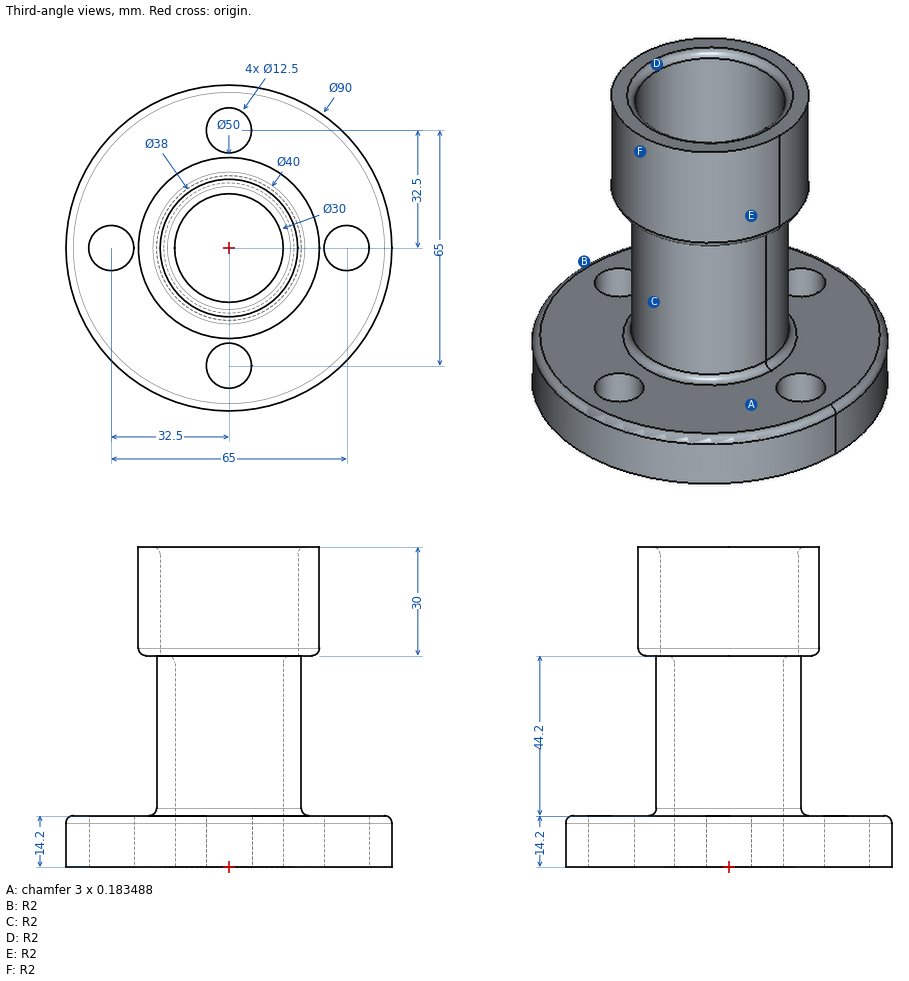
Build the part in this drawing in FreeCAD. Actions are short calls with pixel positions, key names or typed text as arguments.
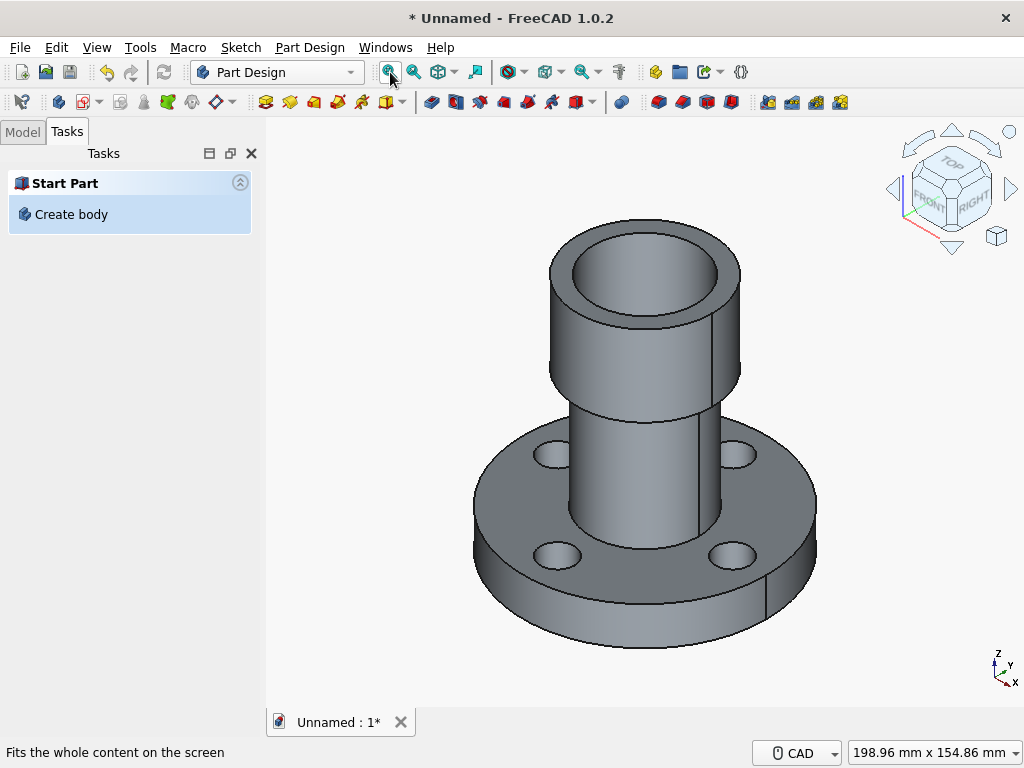
click(492, 549)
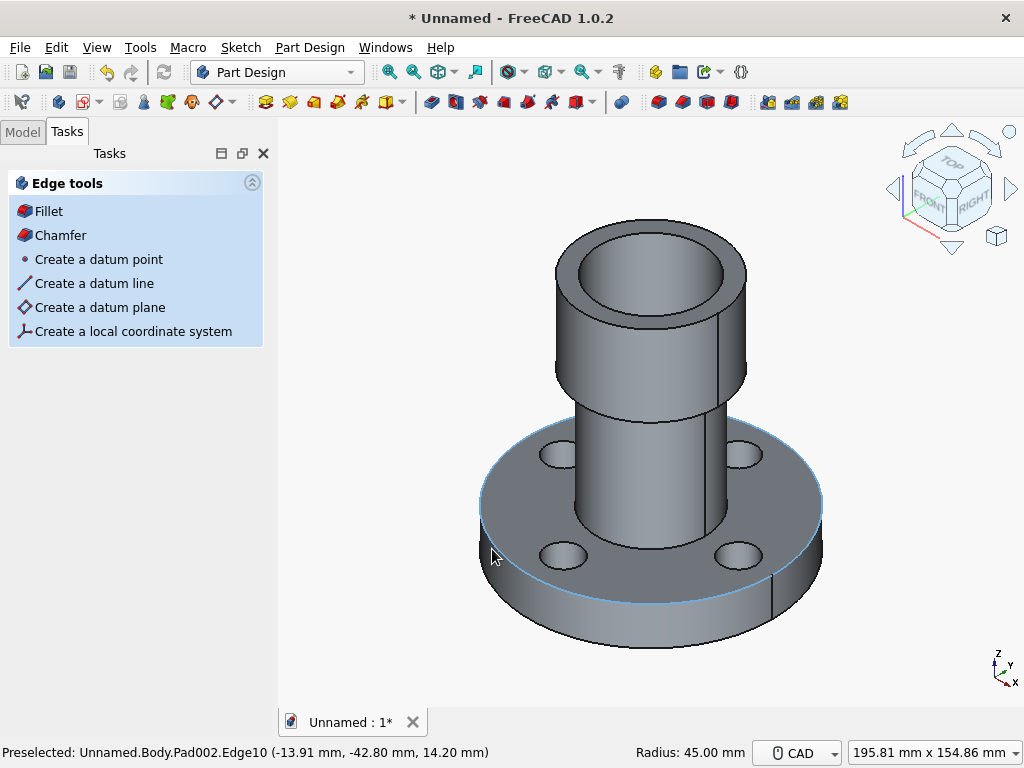
click(660, 102)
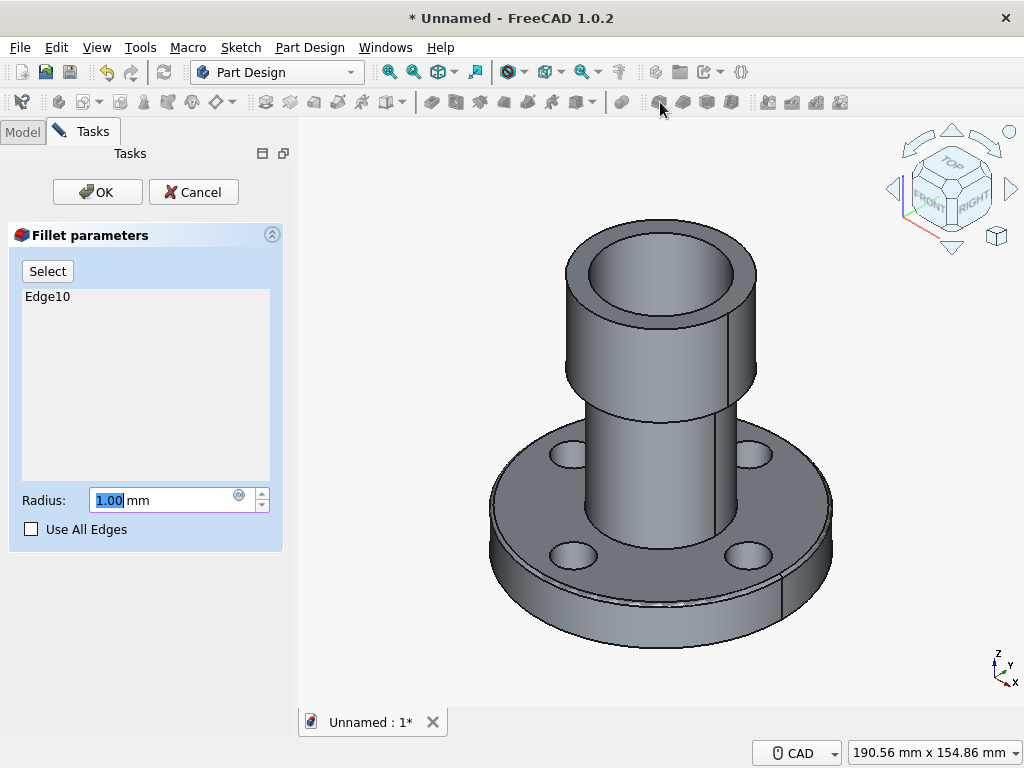
text(2)
key(Tab)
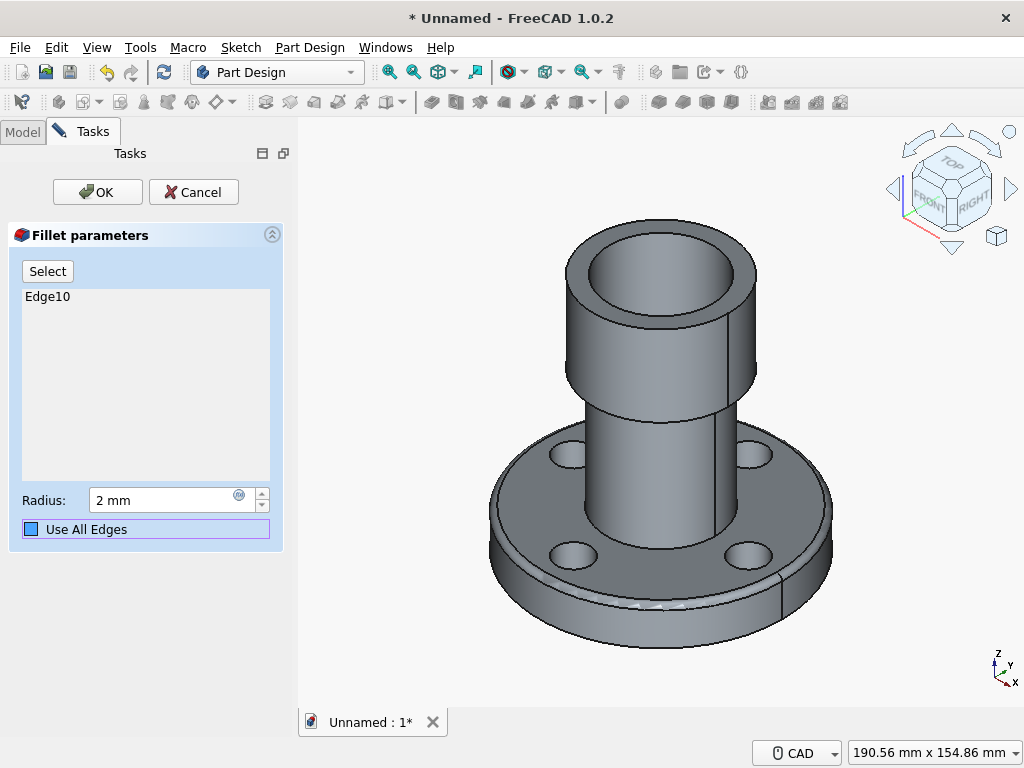
click(98, 192)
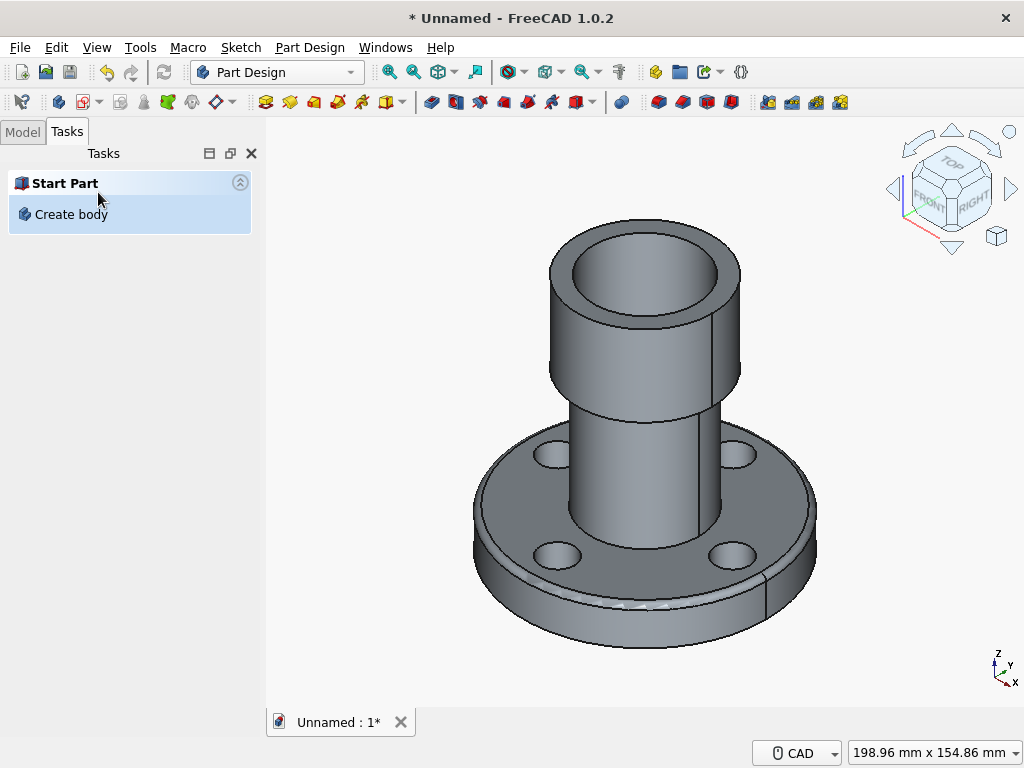
key(2)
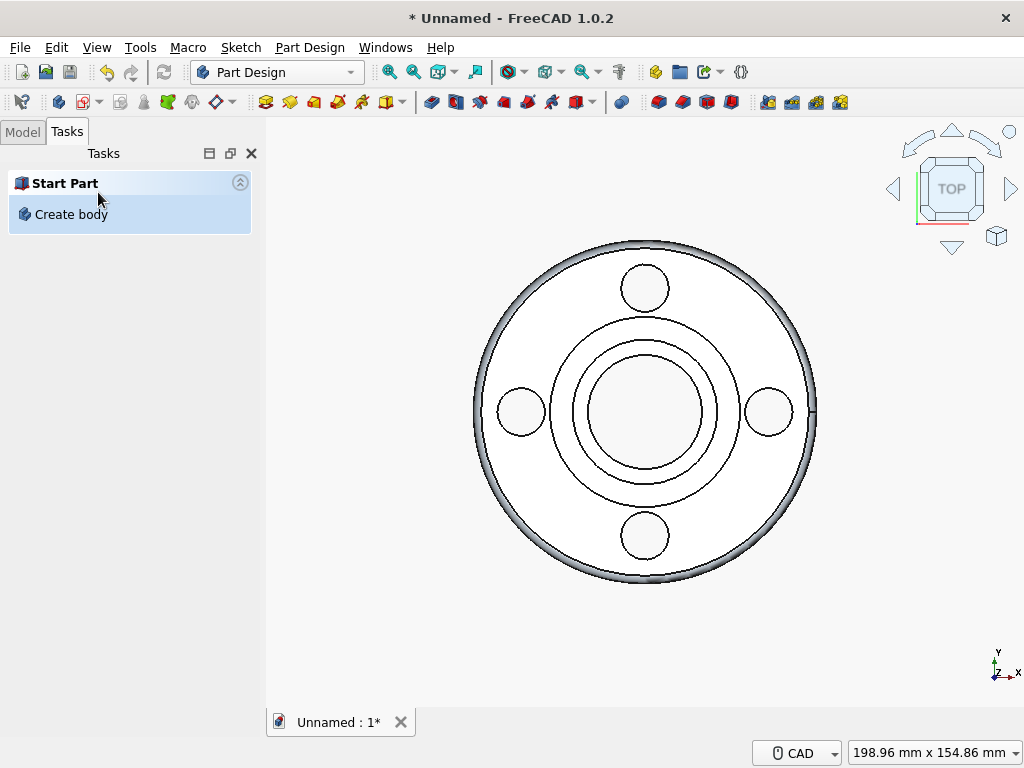
key(0)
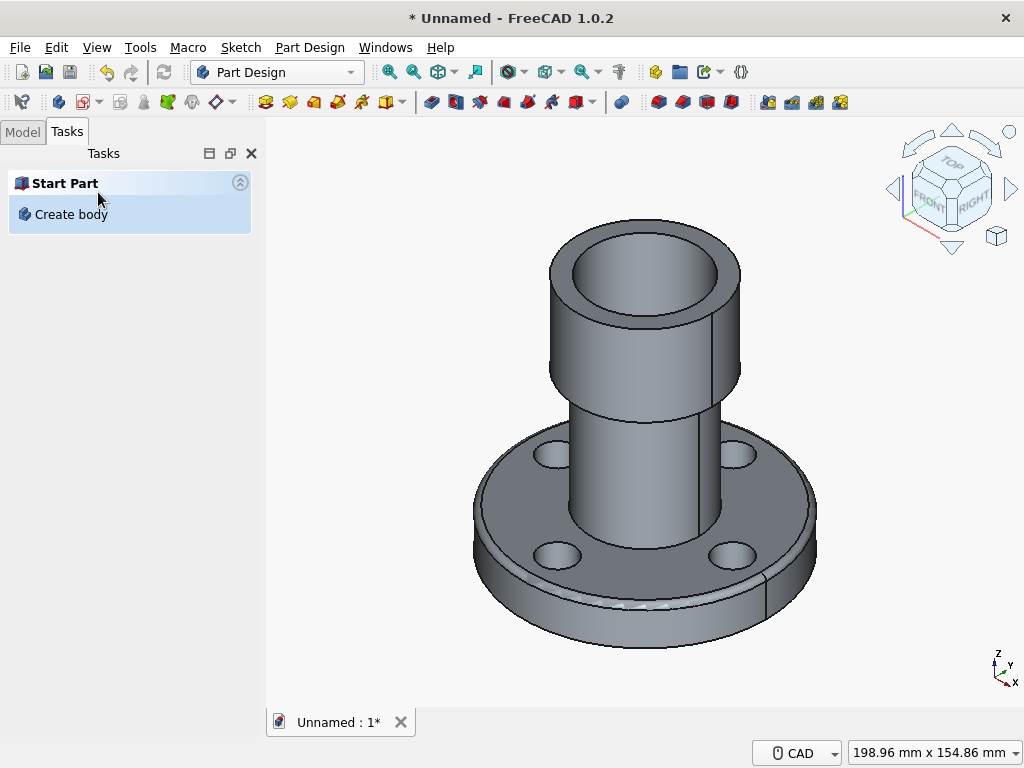
key(1)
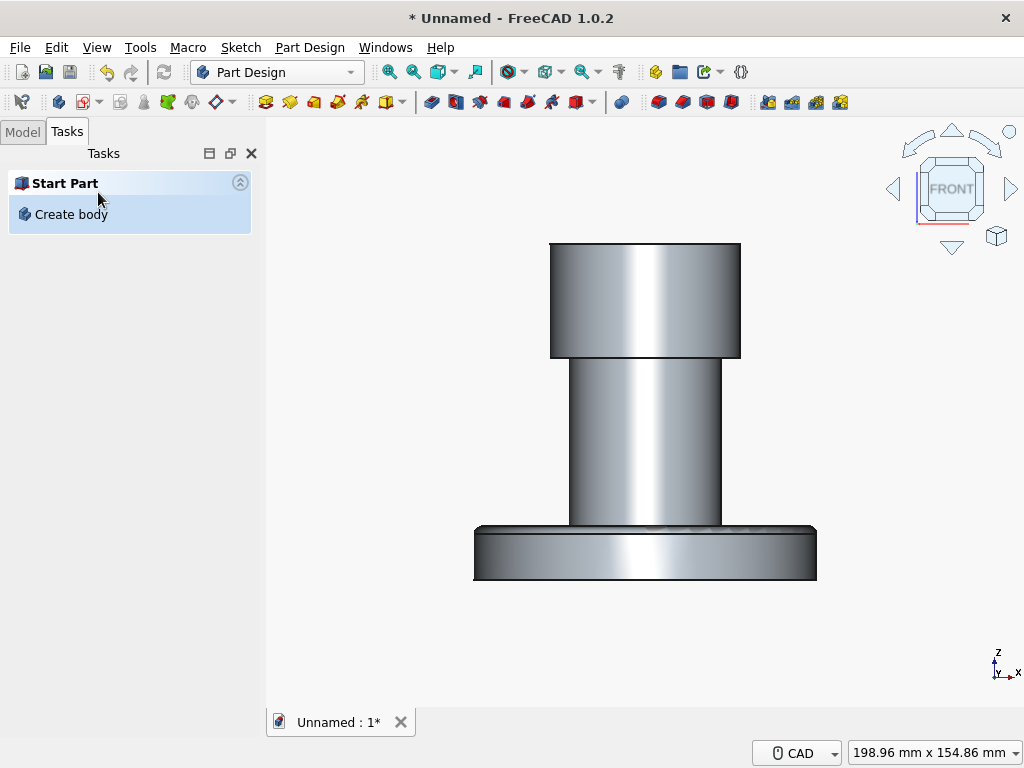
key(3)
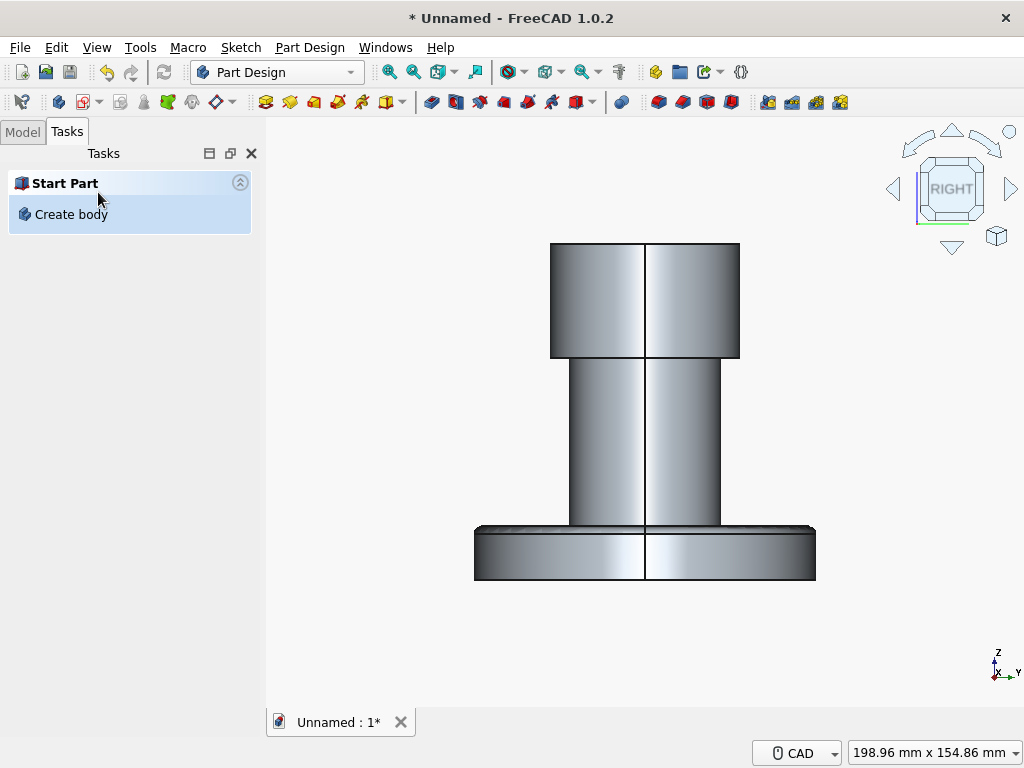
key(5)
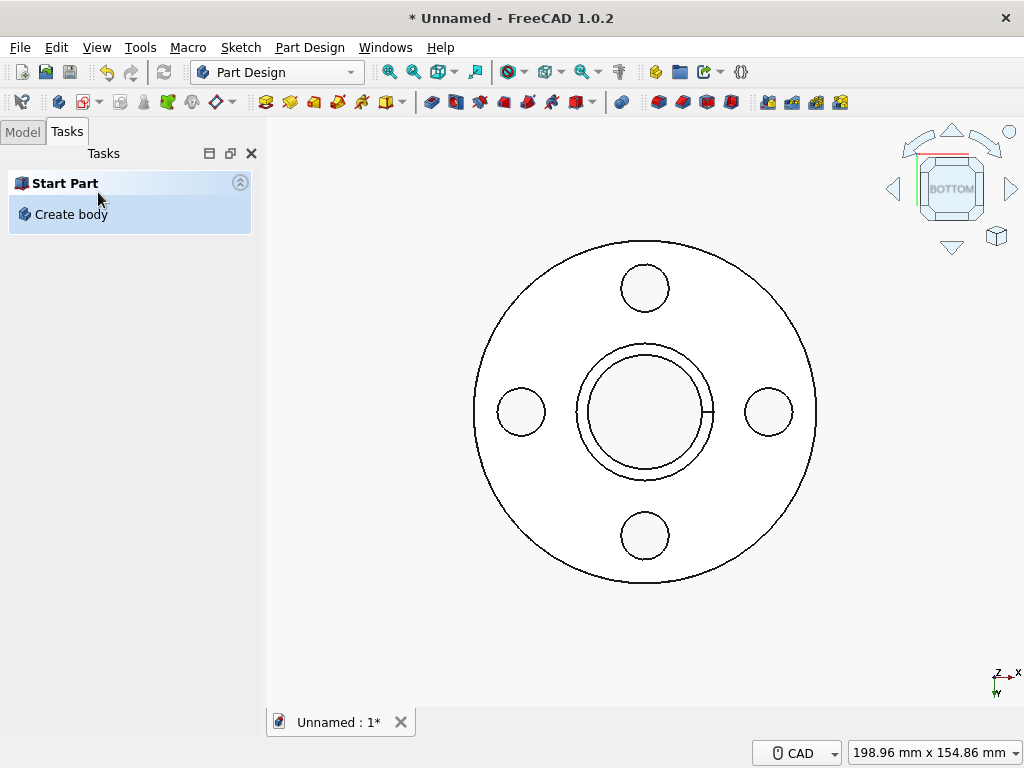
key(4)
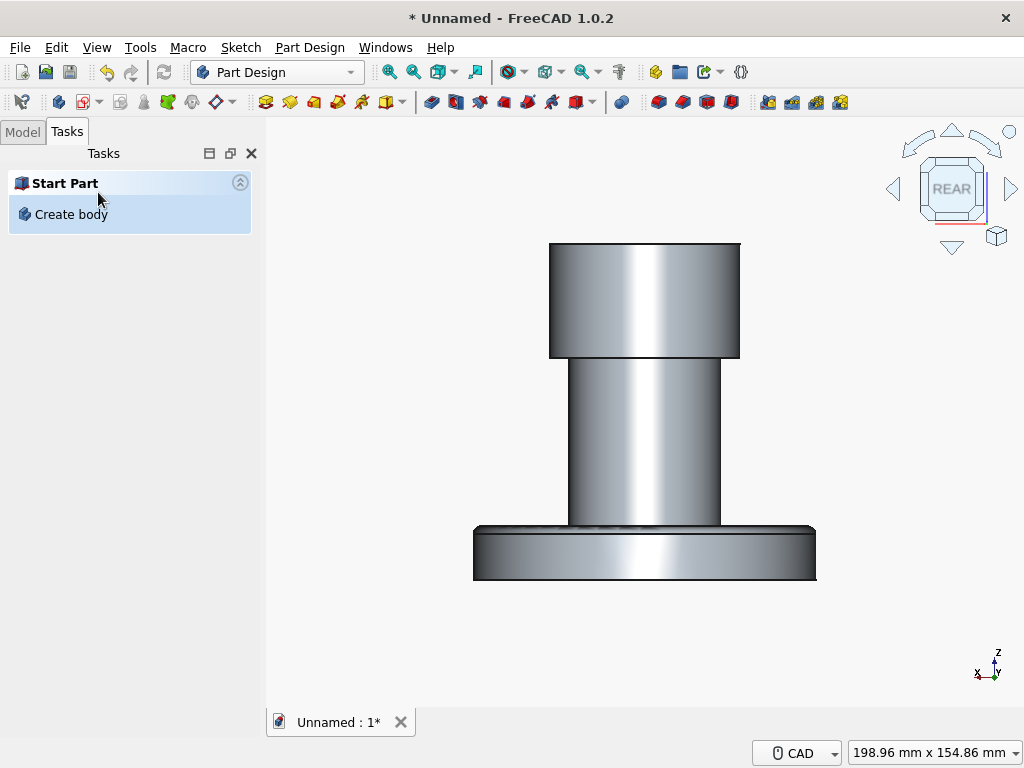
key(6)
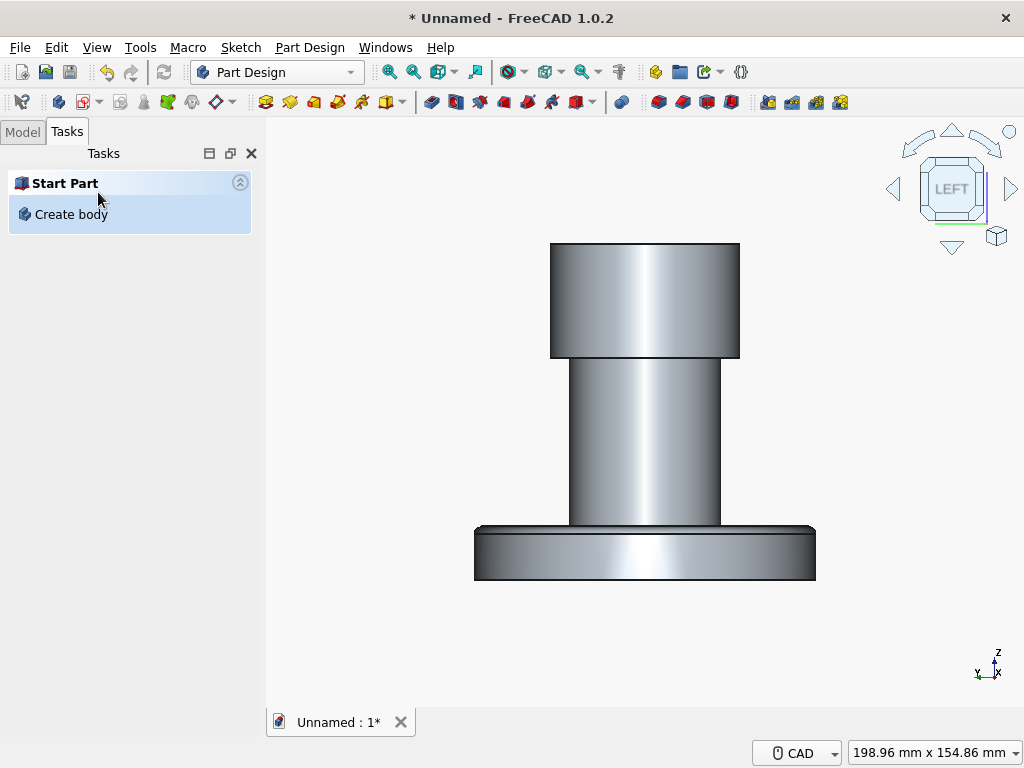
key(v)
key(3)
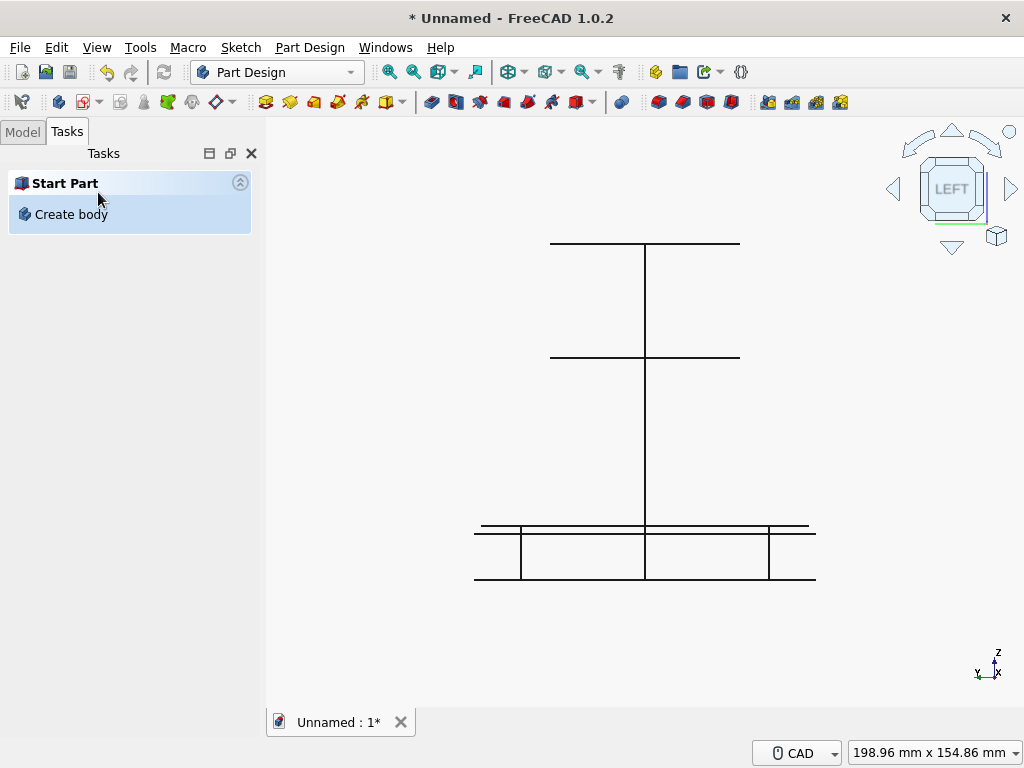
key(0)